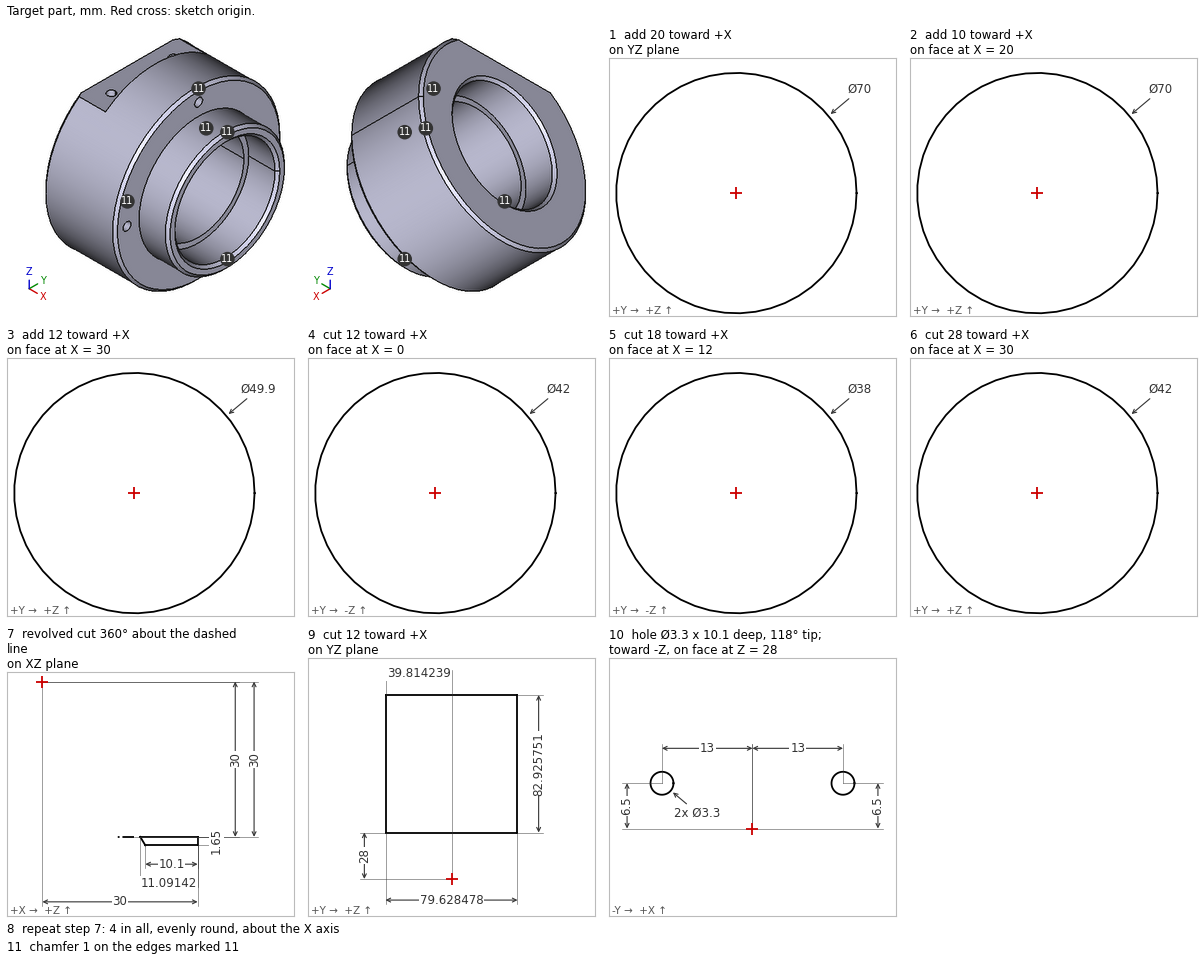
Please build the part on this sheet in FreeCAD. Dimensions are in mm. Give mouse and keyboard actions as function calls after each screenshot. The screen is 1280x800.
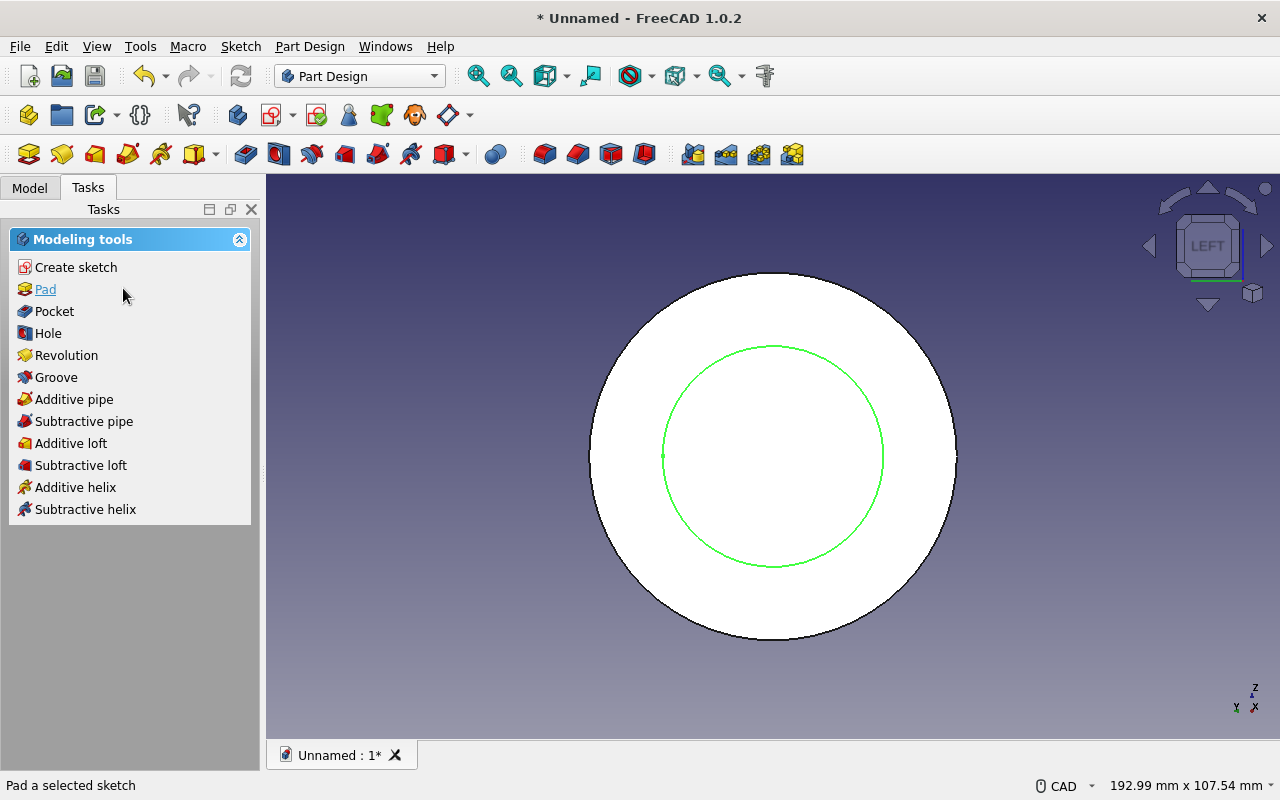
click(246, 154)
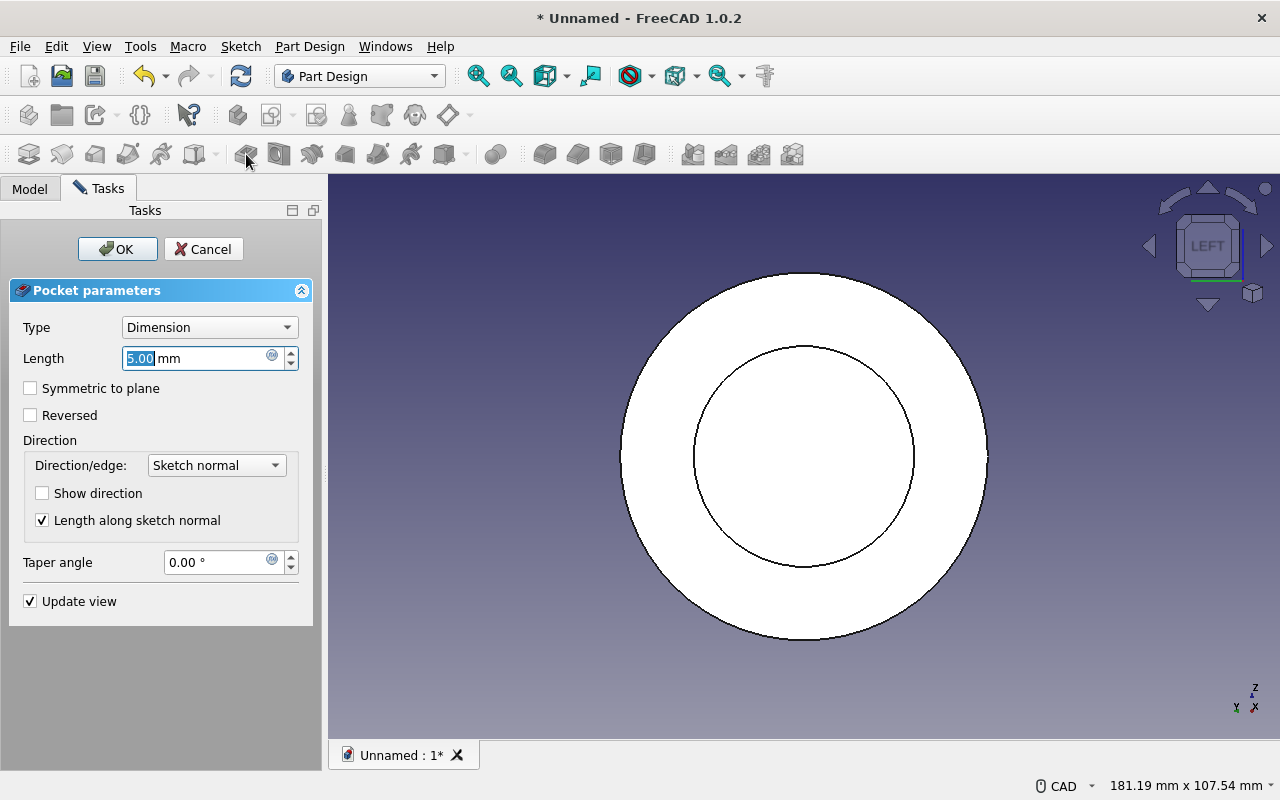
text(12)
key(Tab)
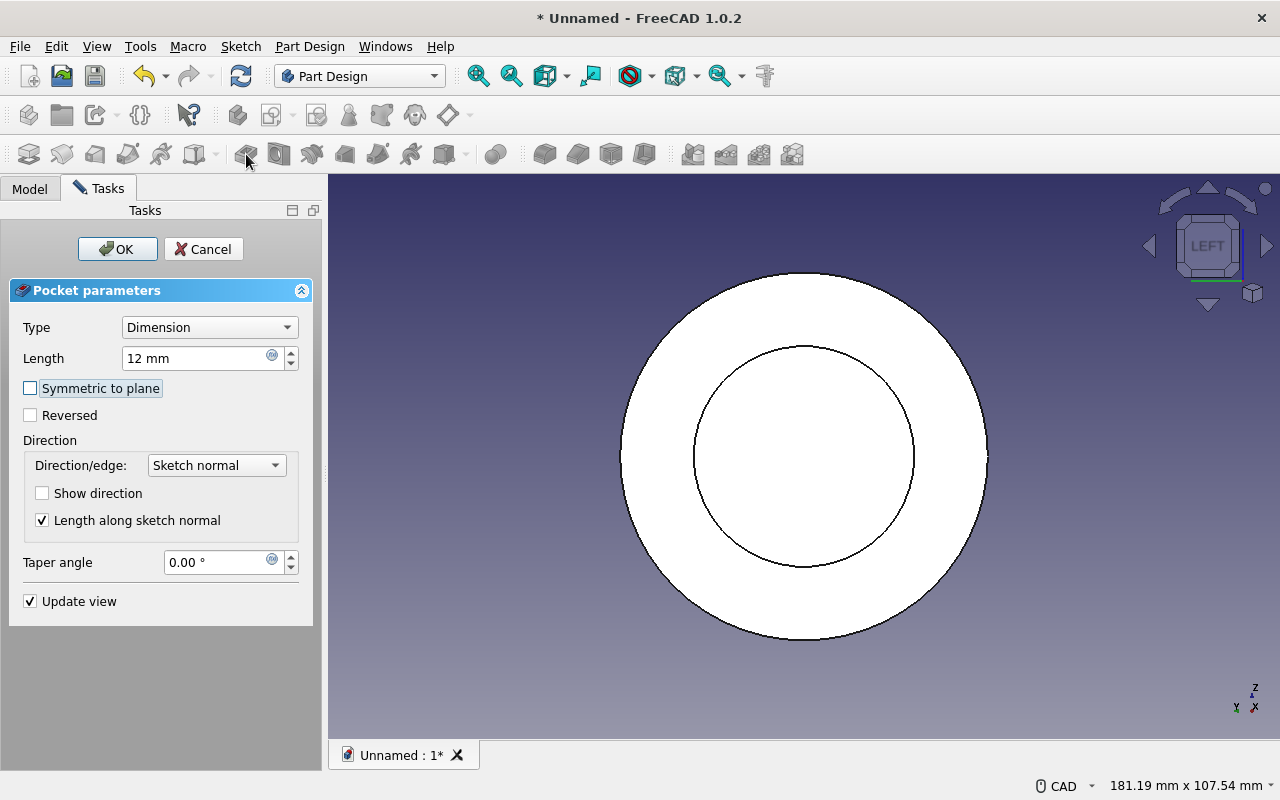
click(118, 249)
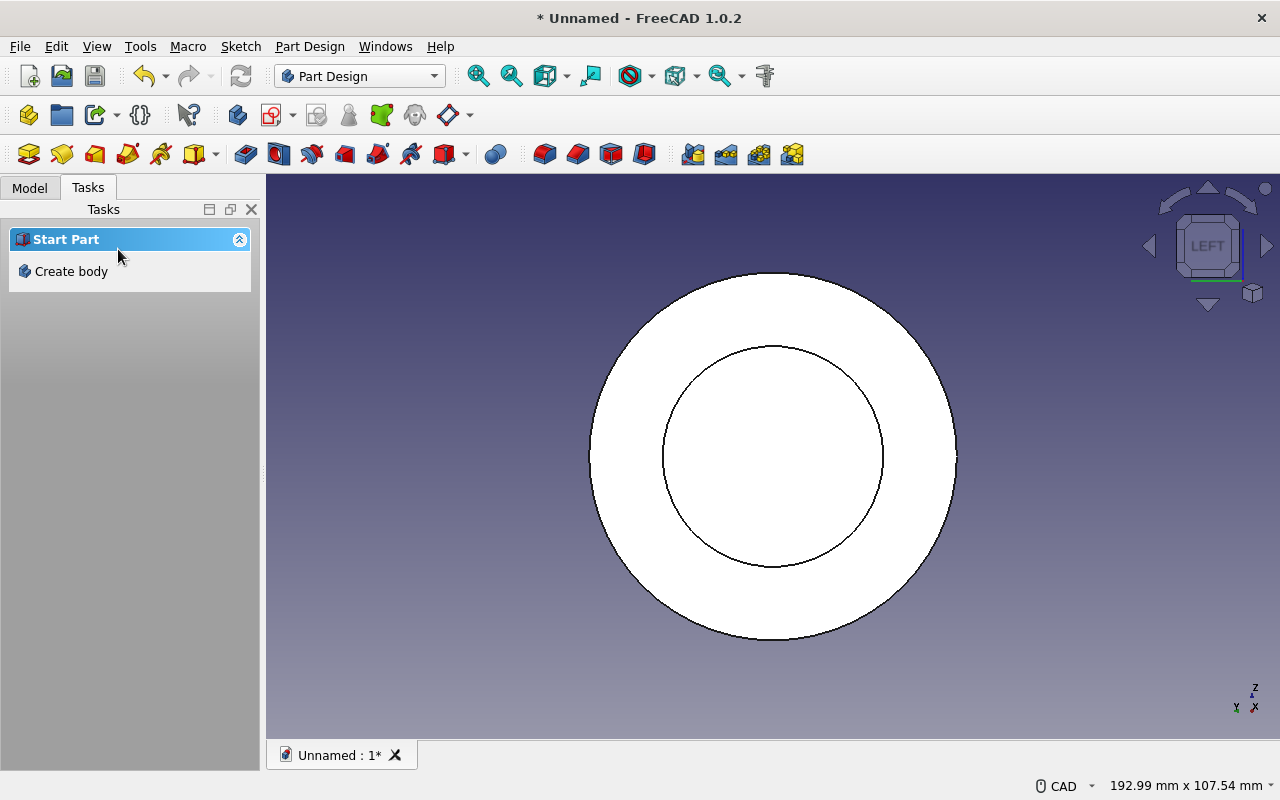
click(773, 455)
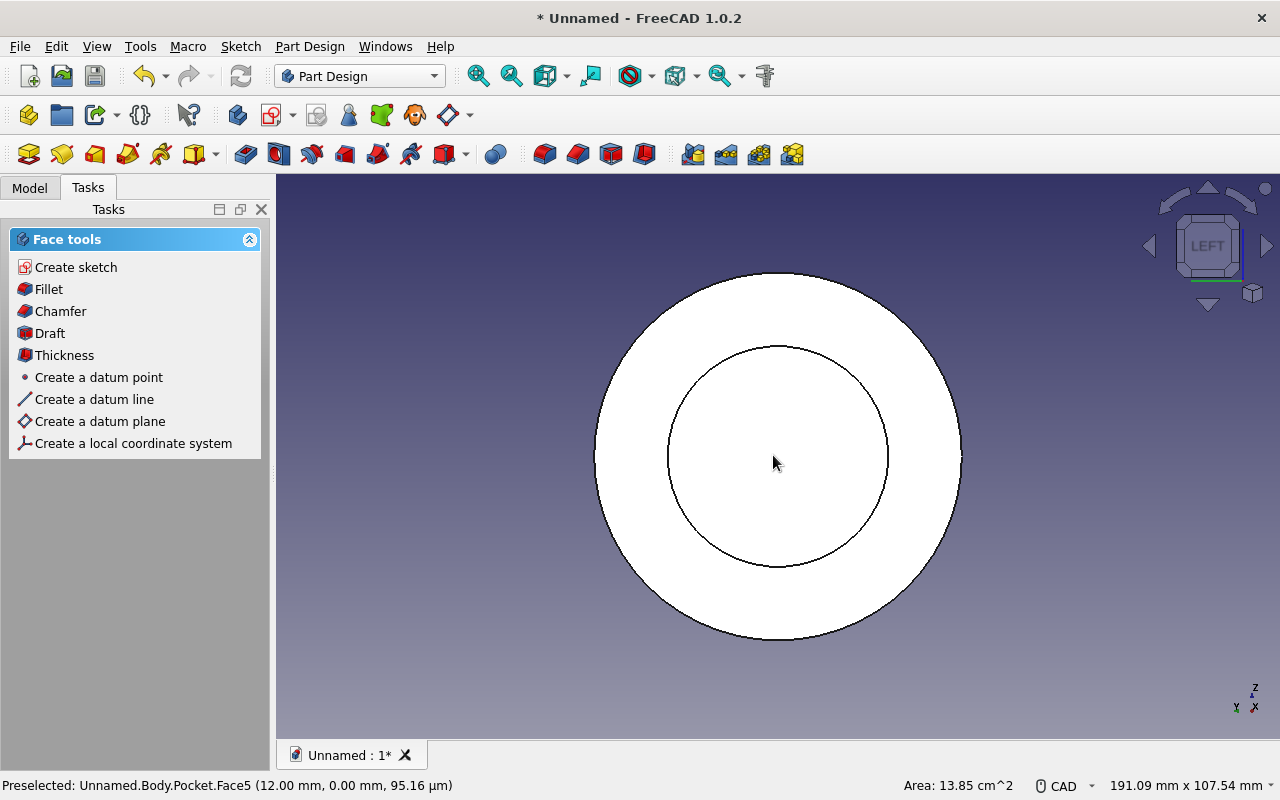
click(270, 116)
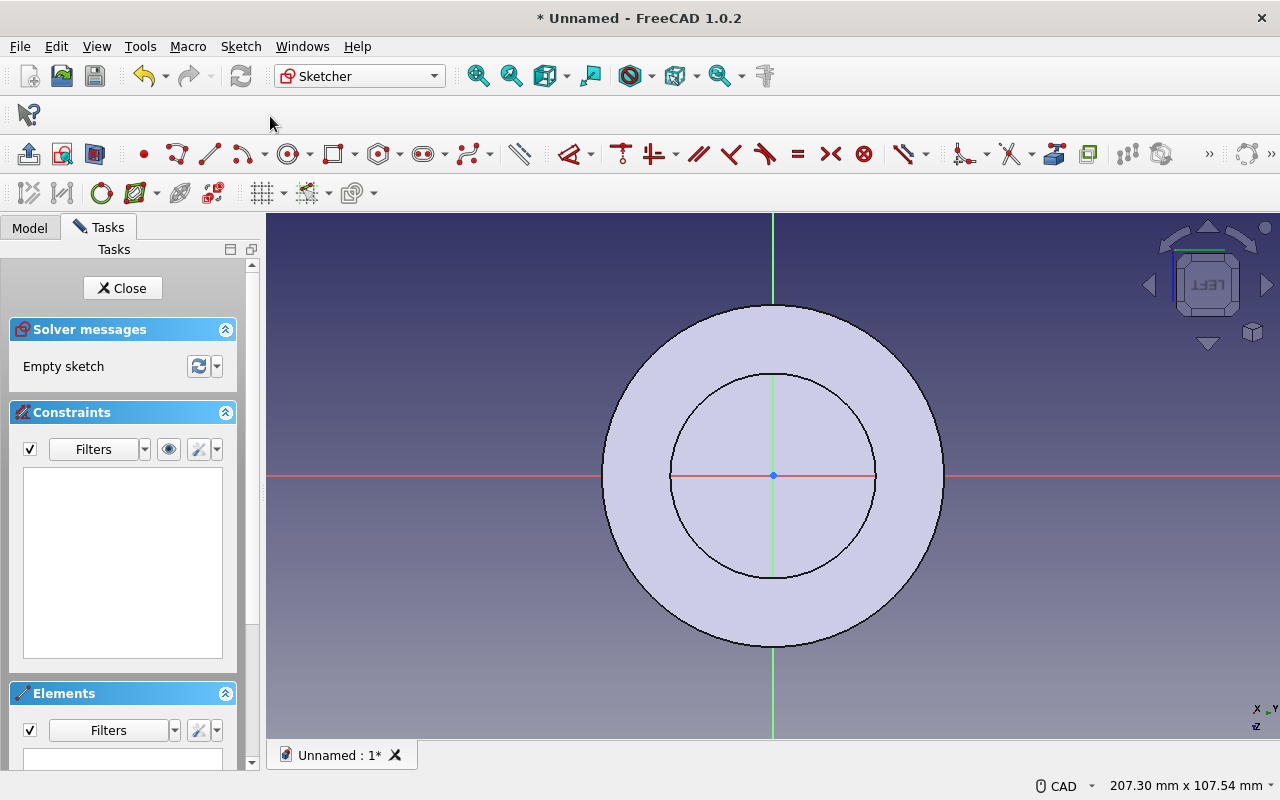
click(95, 154)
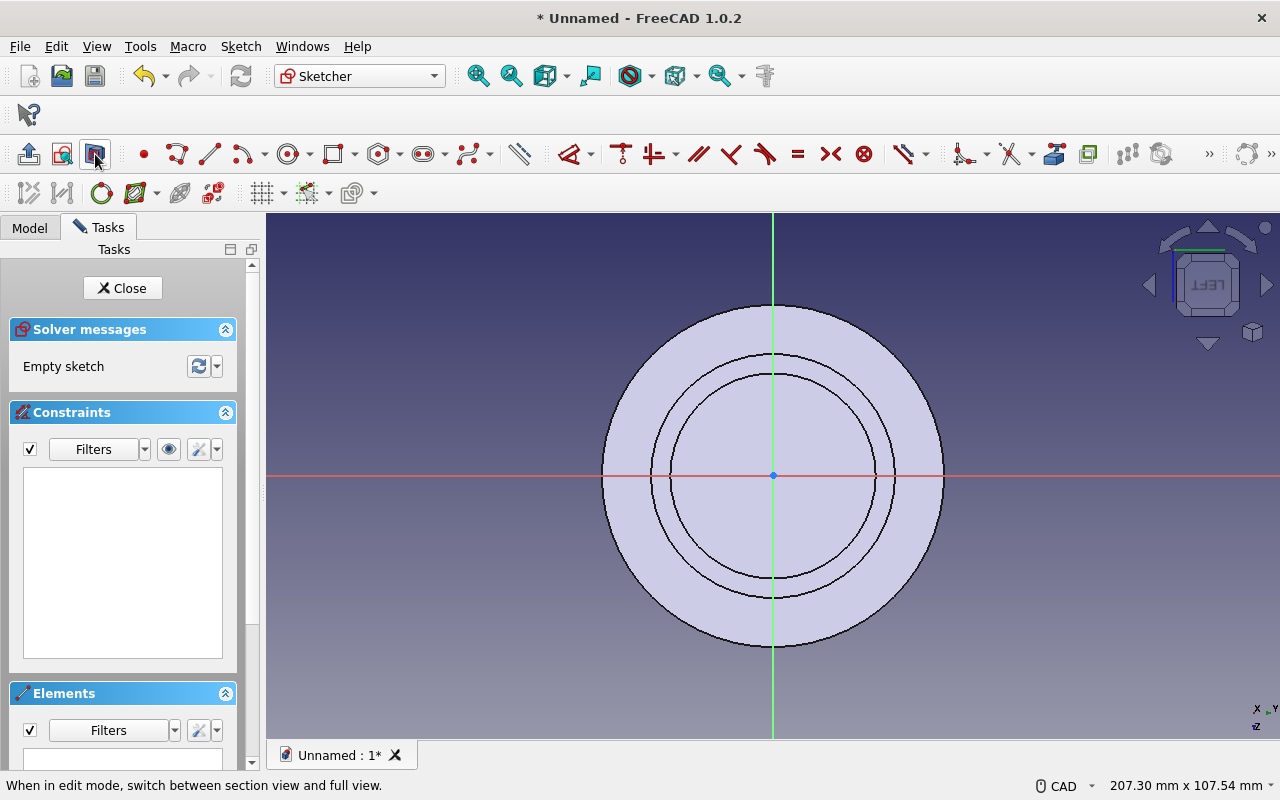
scroll(856, 476, up, 3)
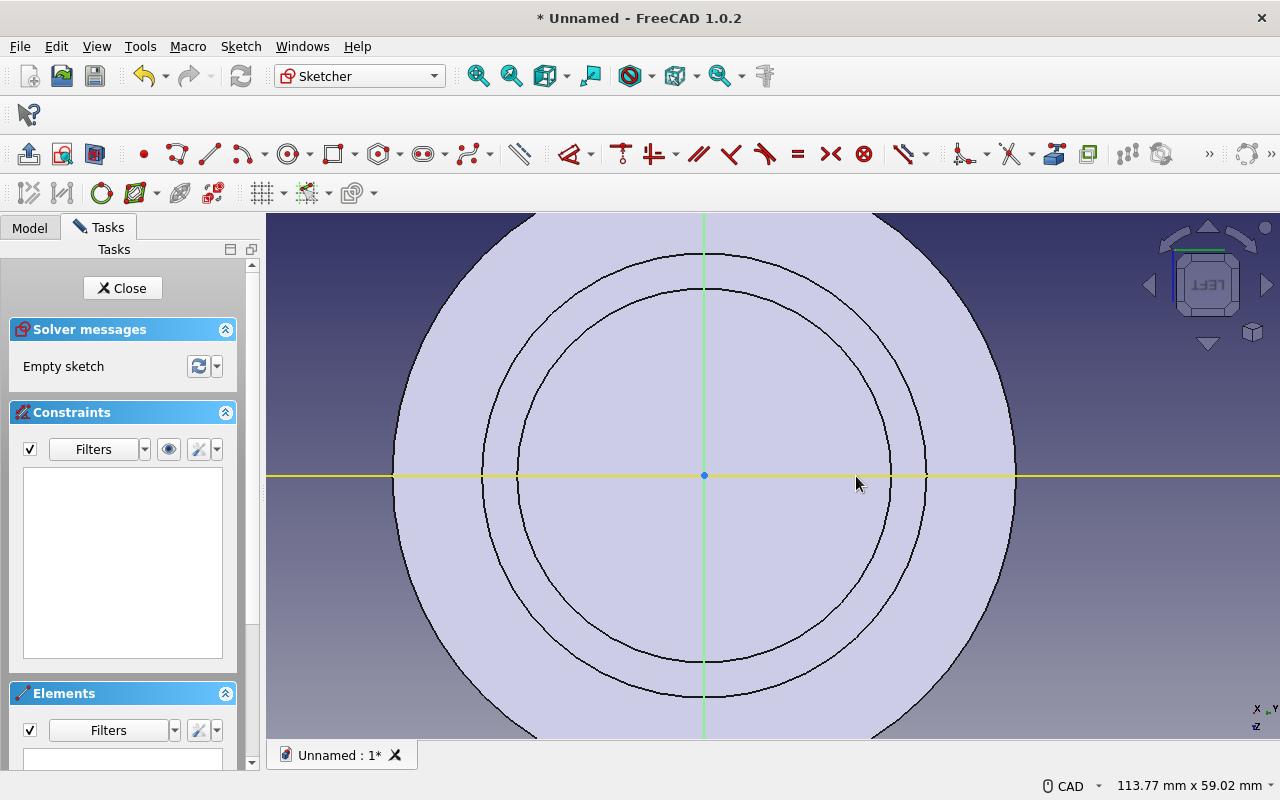
click(288, 154)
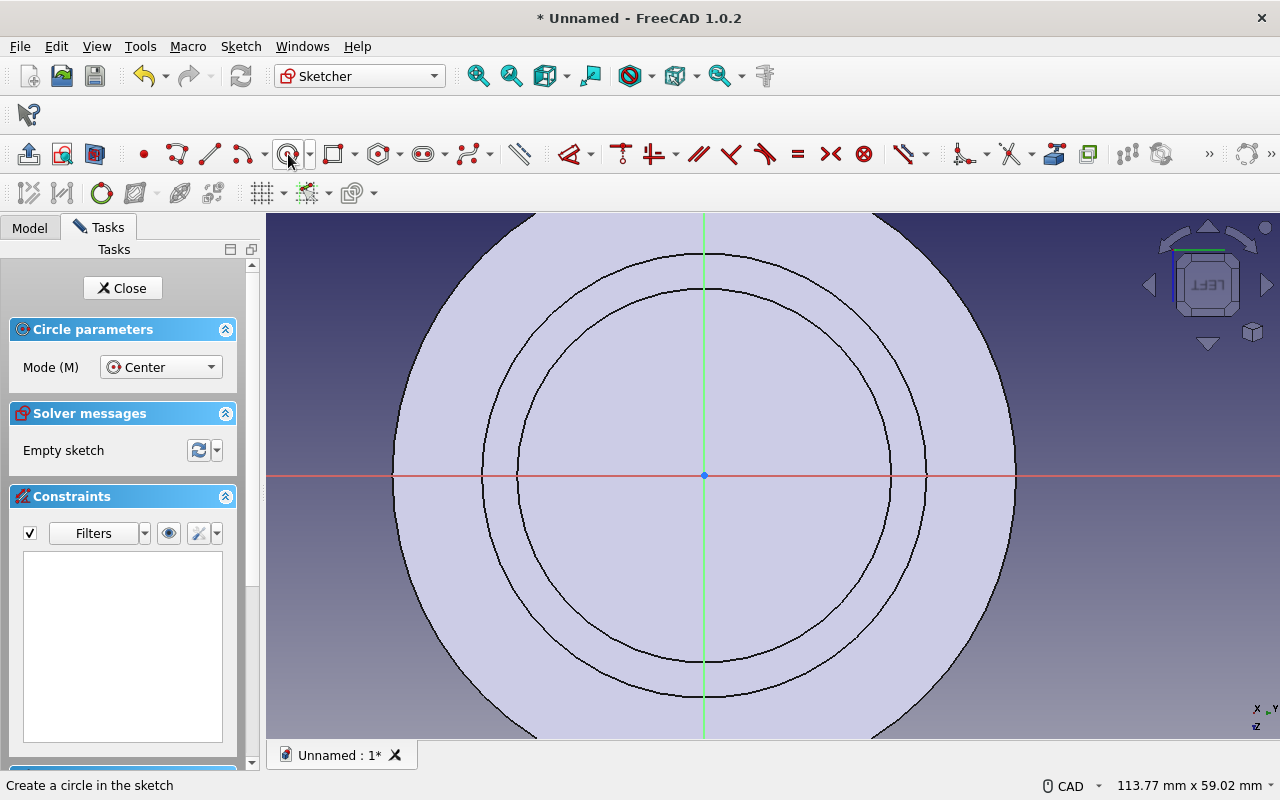
click(704, 476)
move(824, 356)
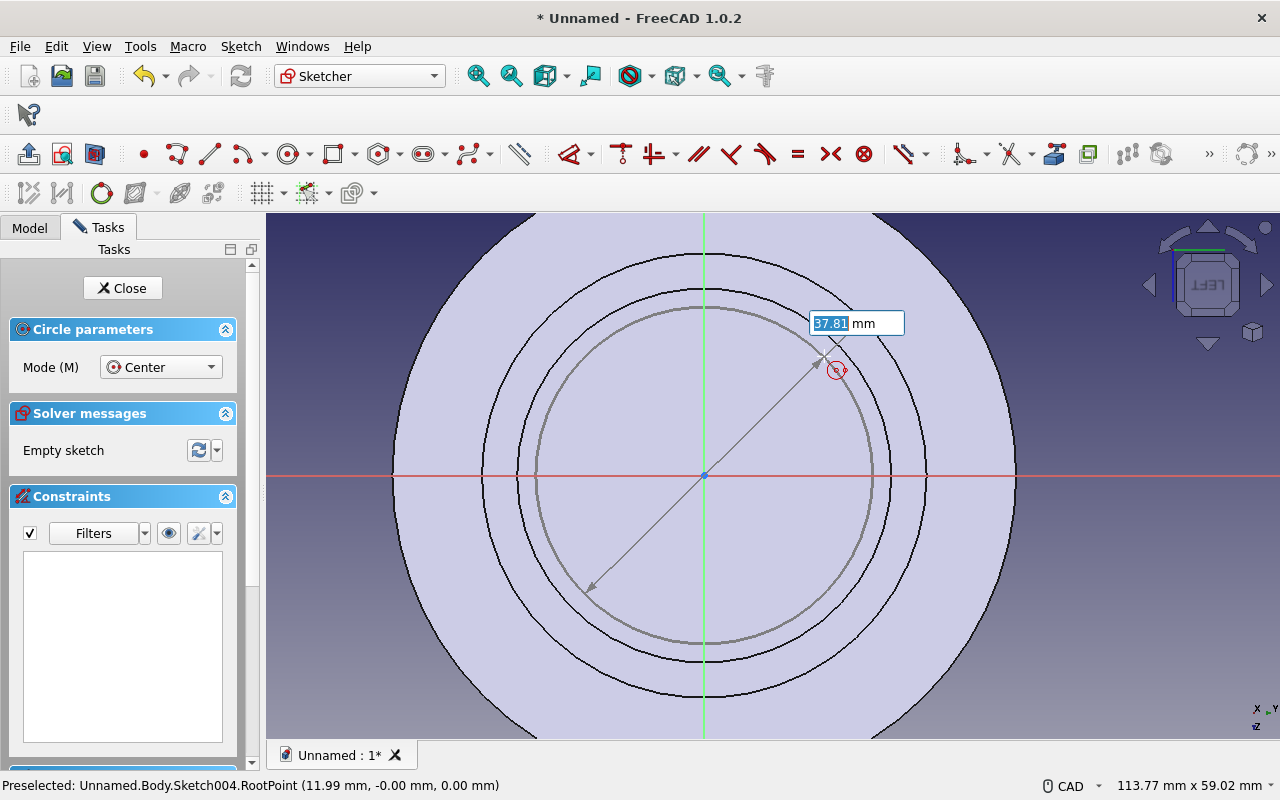
text(38)
key(Return)
key(Escape)